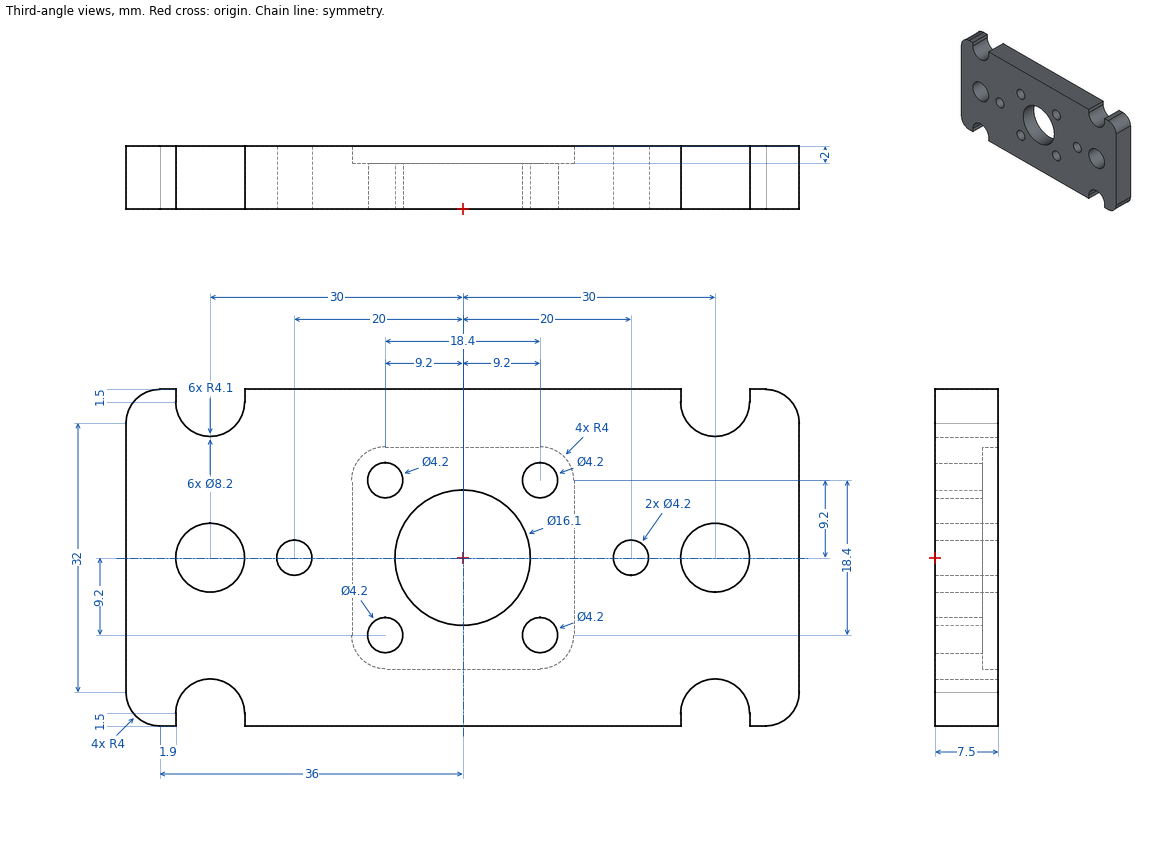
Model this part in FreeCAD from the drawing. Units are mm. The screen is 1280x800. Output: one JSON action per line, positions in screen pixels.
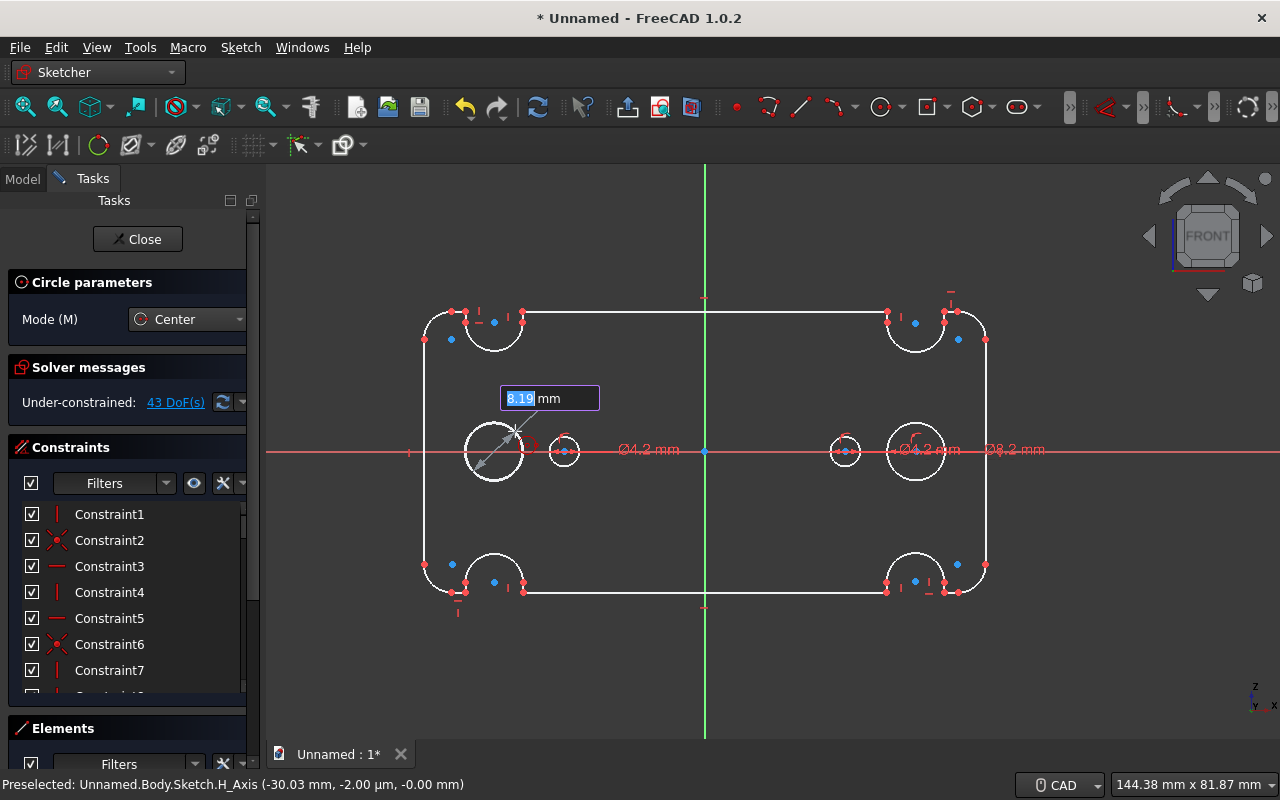
{"action": "type", "text": "8.2"}
{"action": "key", "text": "Return"}
{"action": "key", "text": "Escape"}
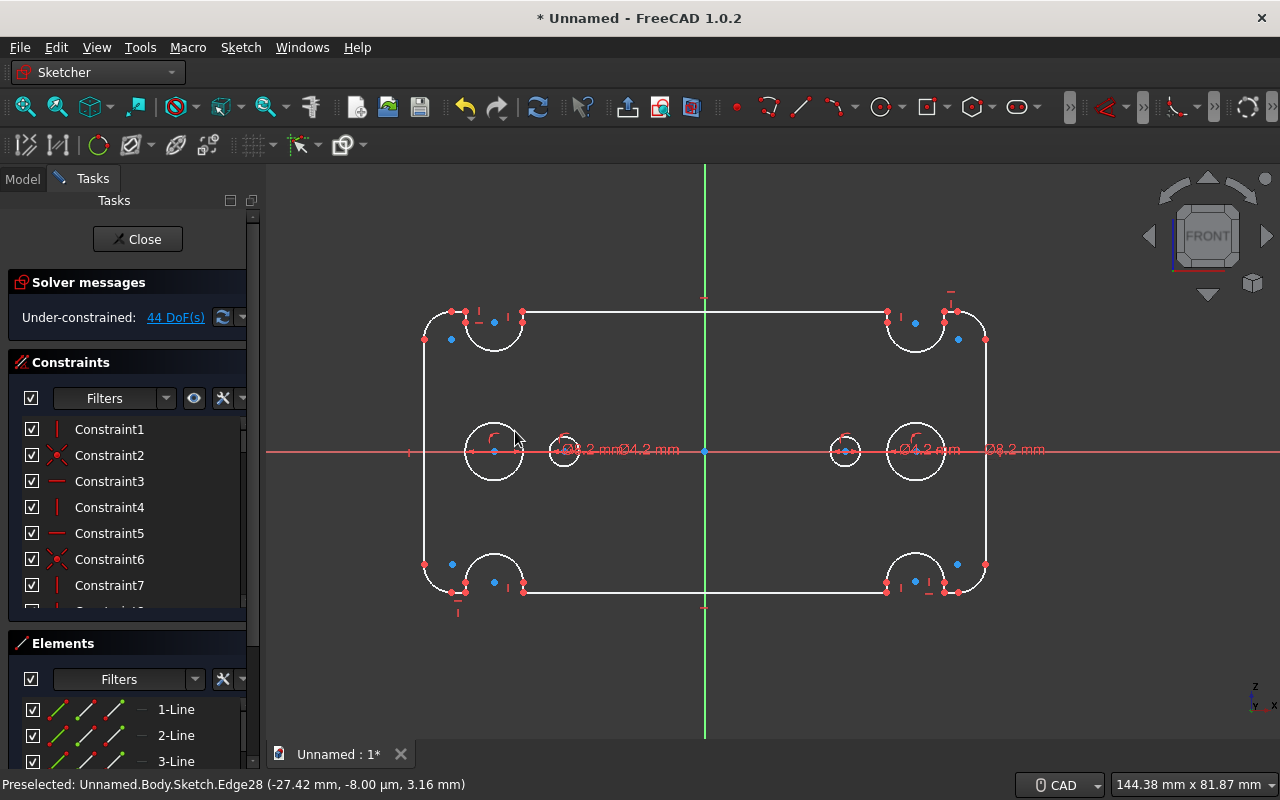
{"action": "scroll", "coordinate": [466, 588], "scroll_direction": "up", "scroll_amount": 6}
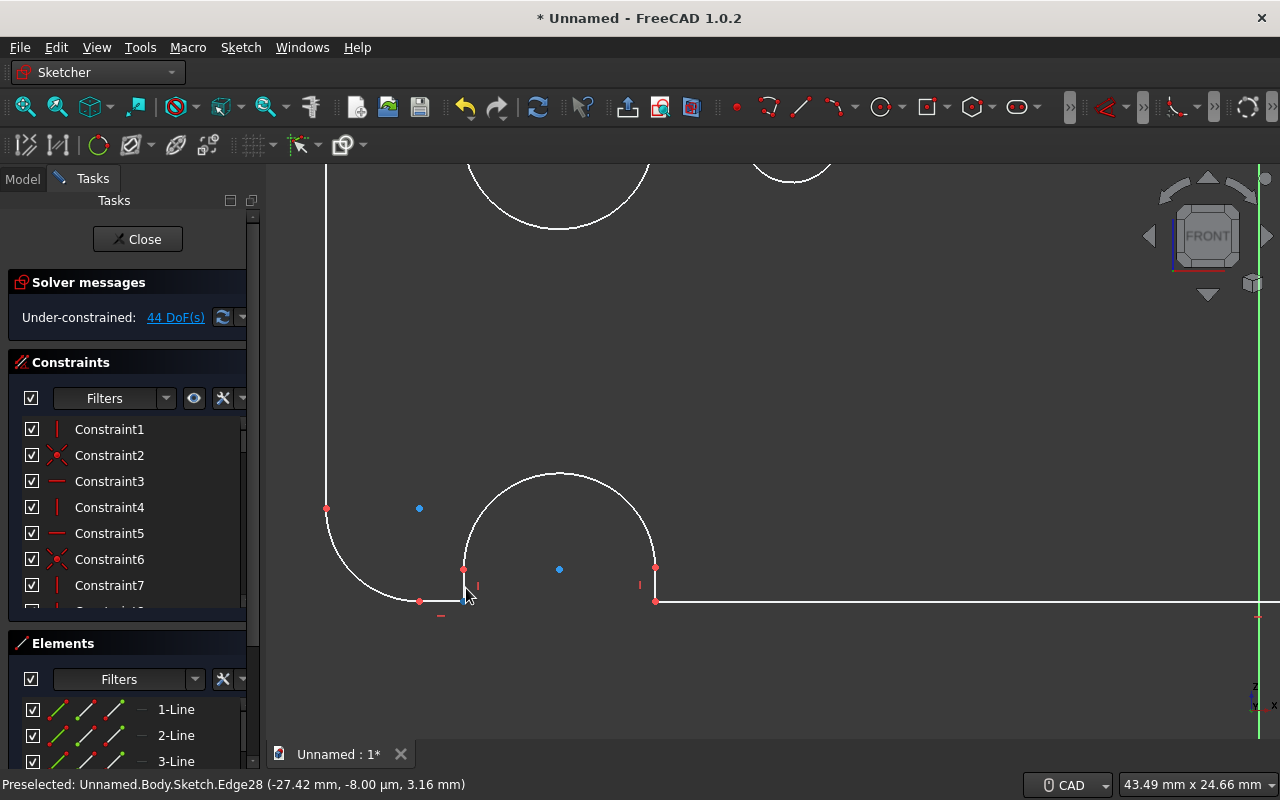
{"action": "left_click", "coordinate": [464, 585]}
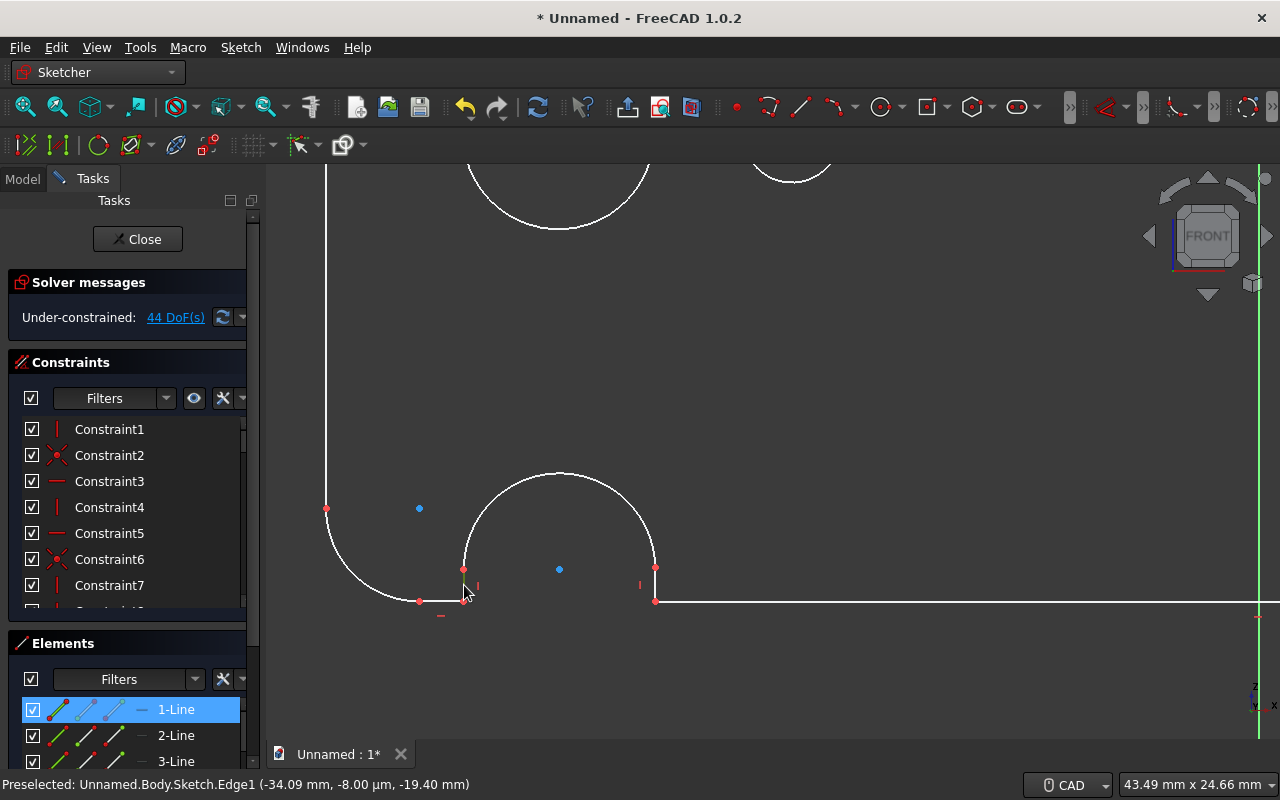
{"action": "scroll", "coordinate": [466, 589], "scroll_direction": "down", "scroll_amount": 6}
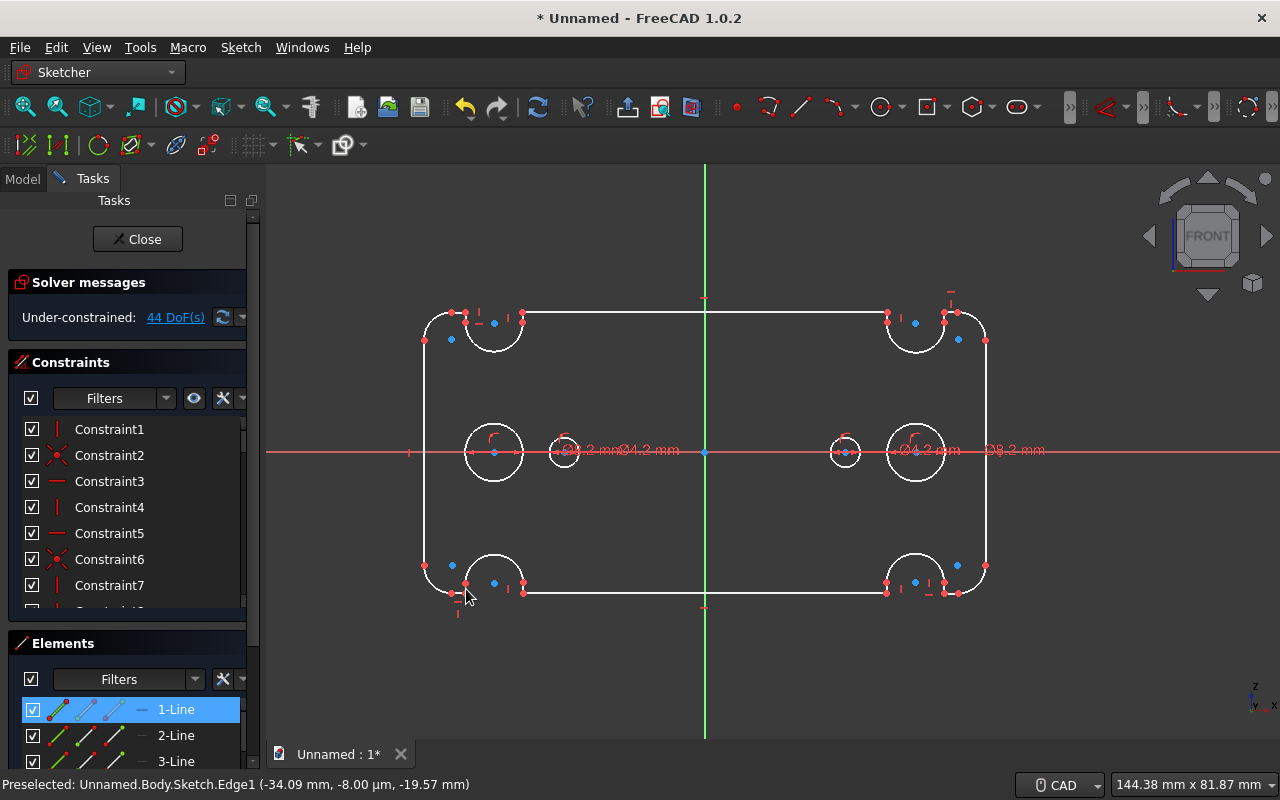
{"action": "left_click", "coordinate": [511, 560]}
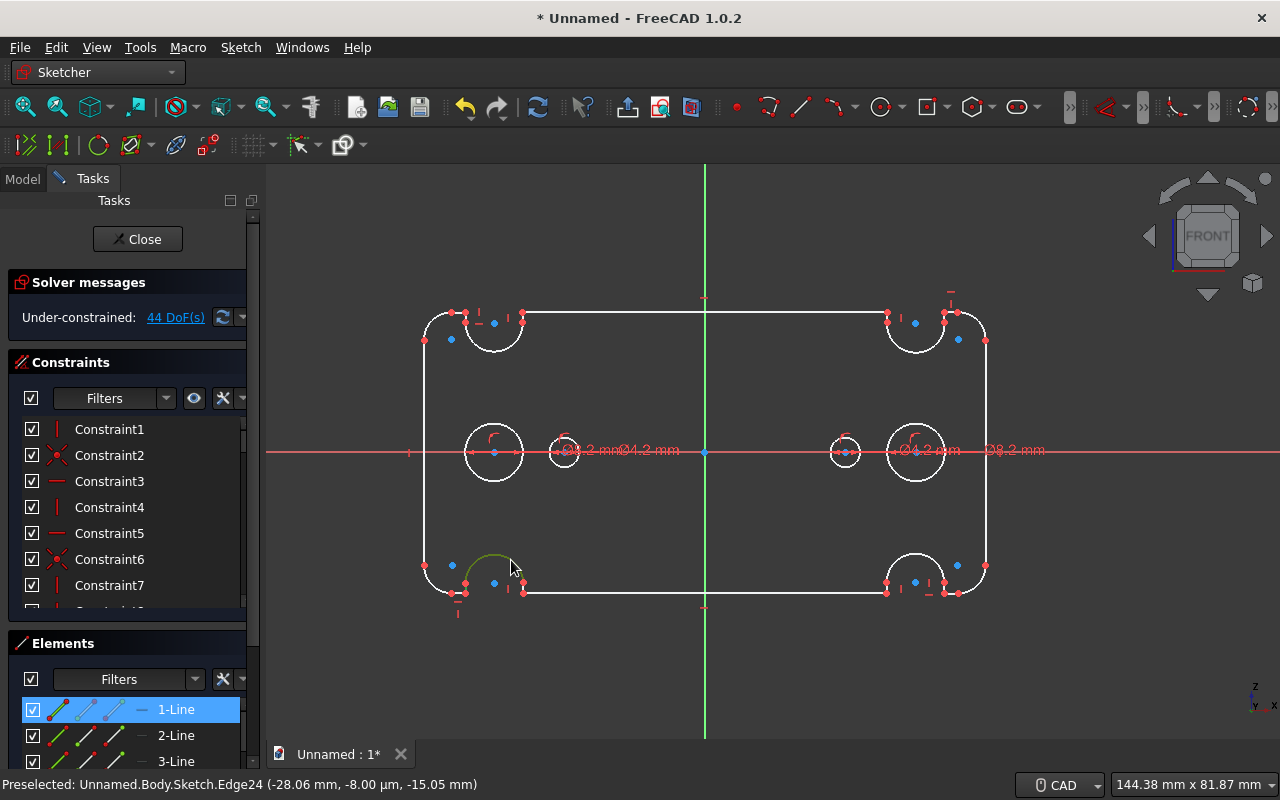
{"action": "key", "text": "t"}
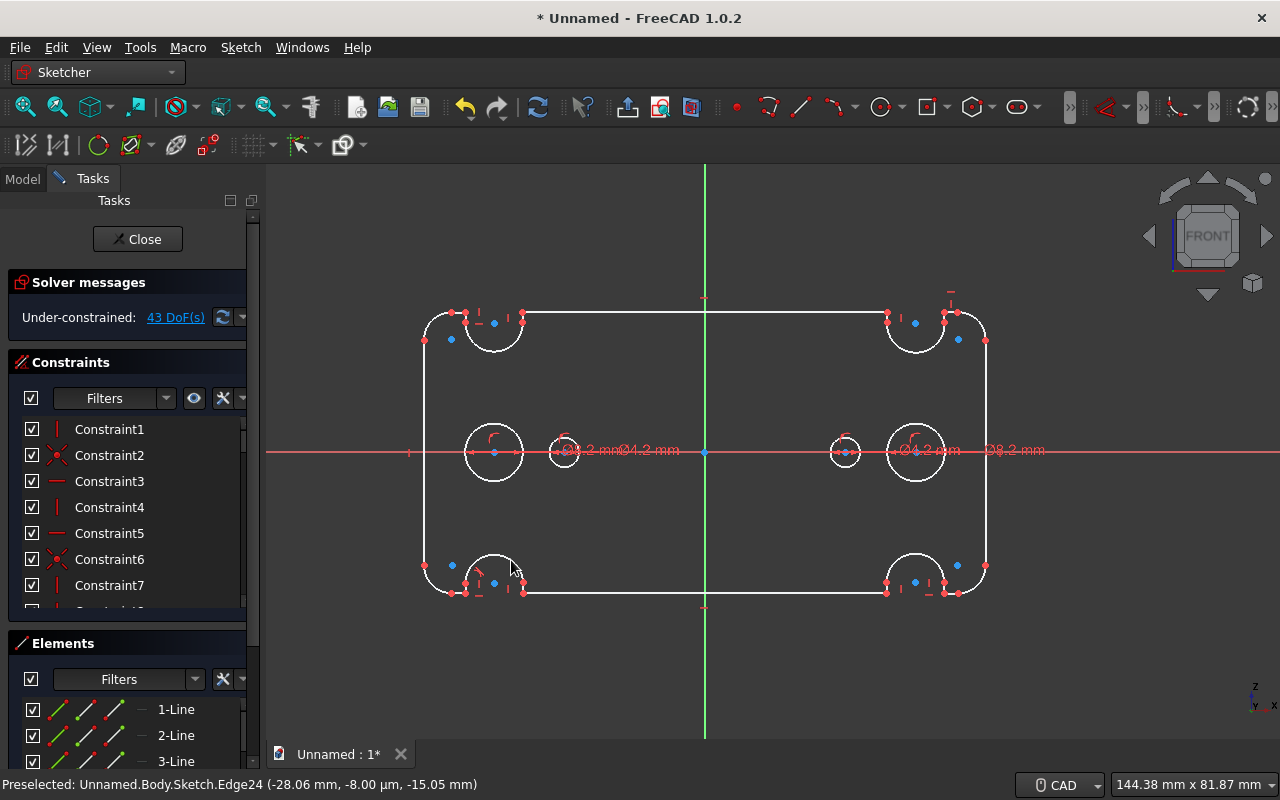
{"action": "scroll", "coordinate": [459, 593], "scroll_direction": "up", "scroll_amount": 4}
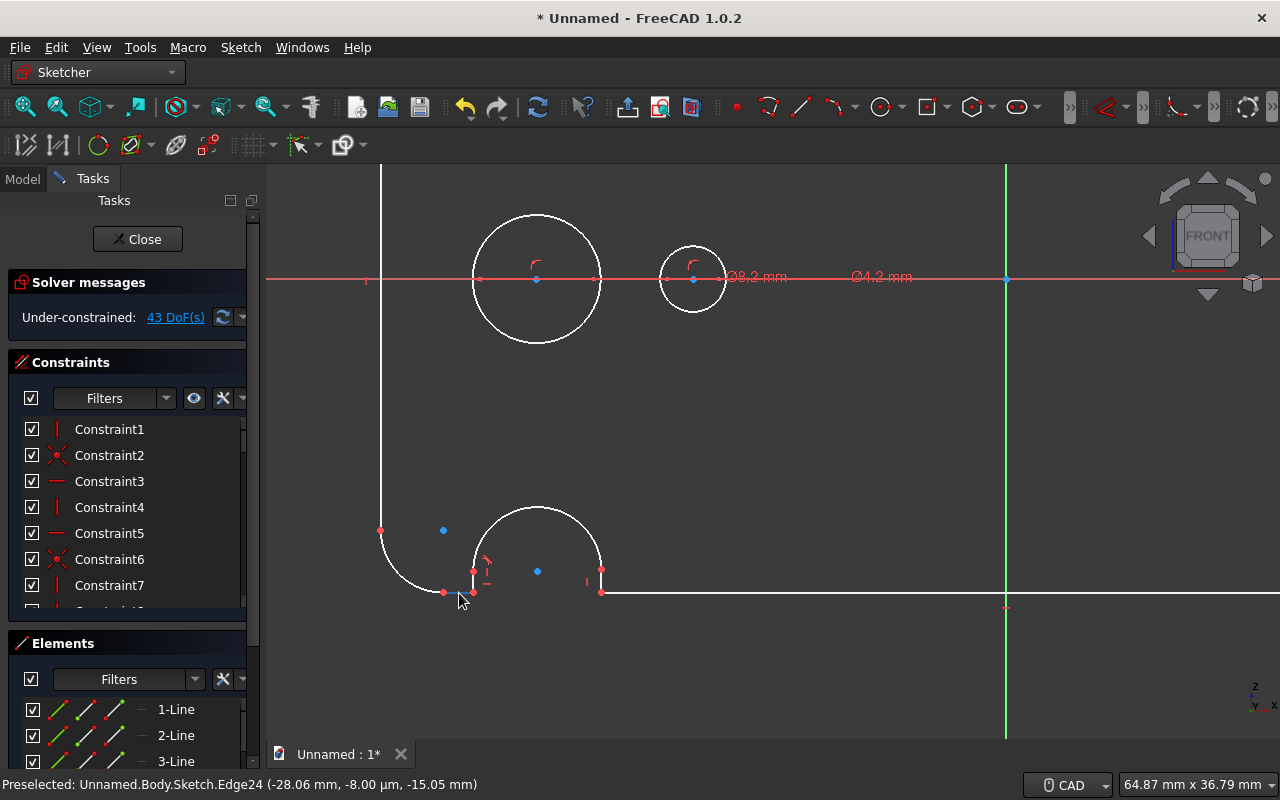
{"action": "left_click", "coordinate": [458, 593]}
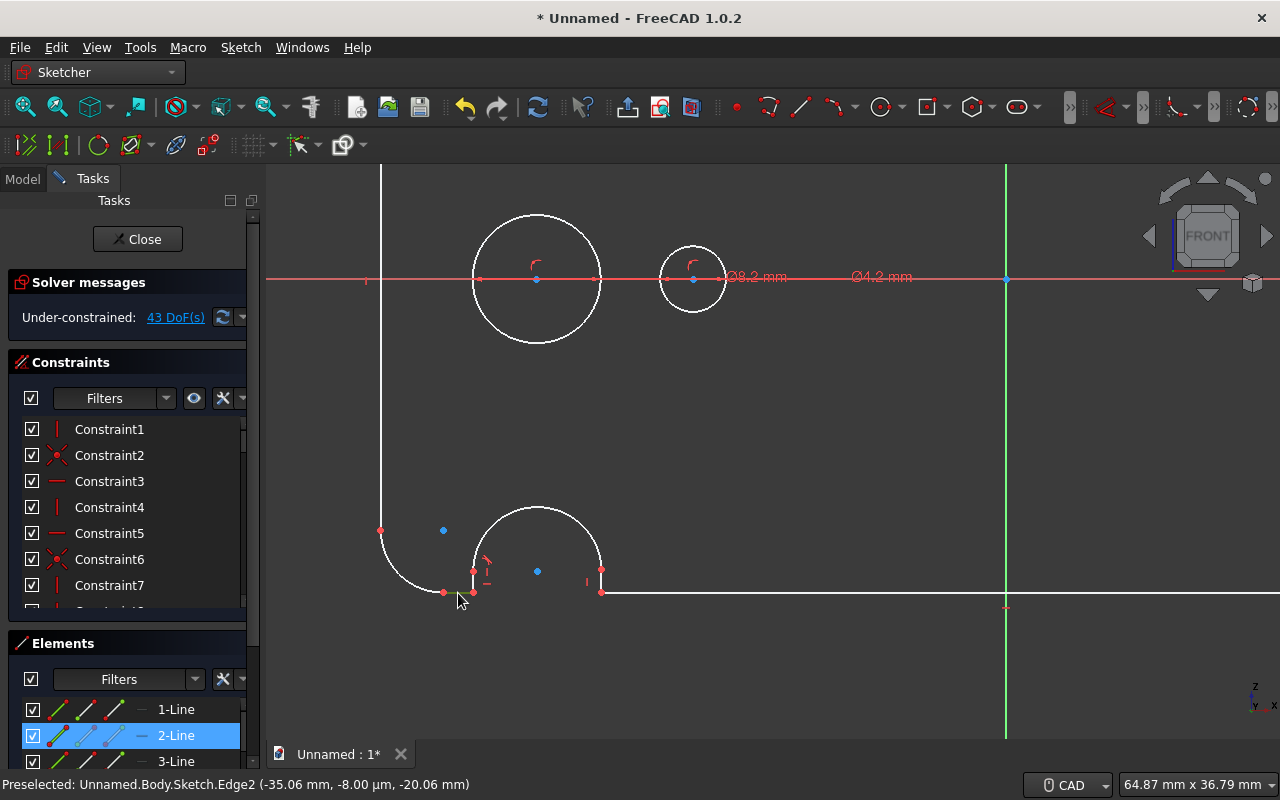
{"action": "left_click", "coordinate": [388, 559]}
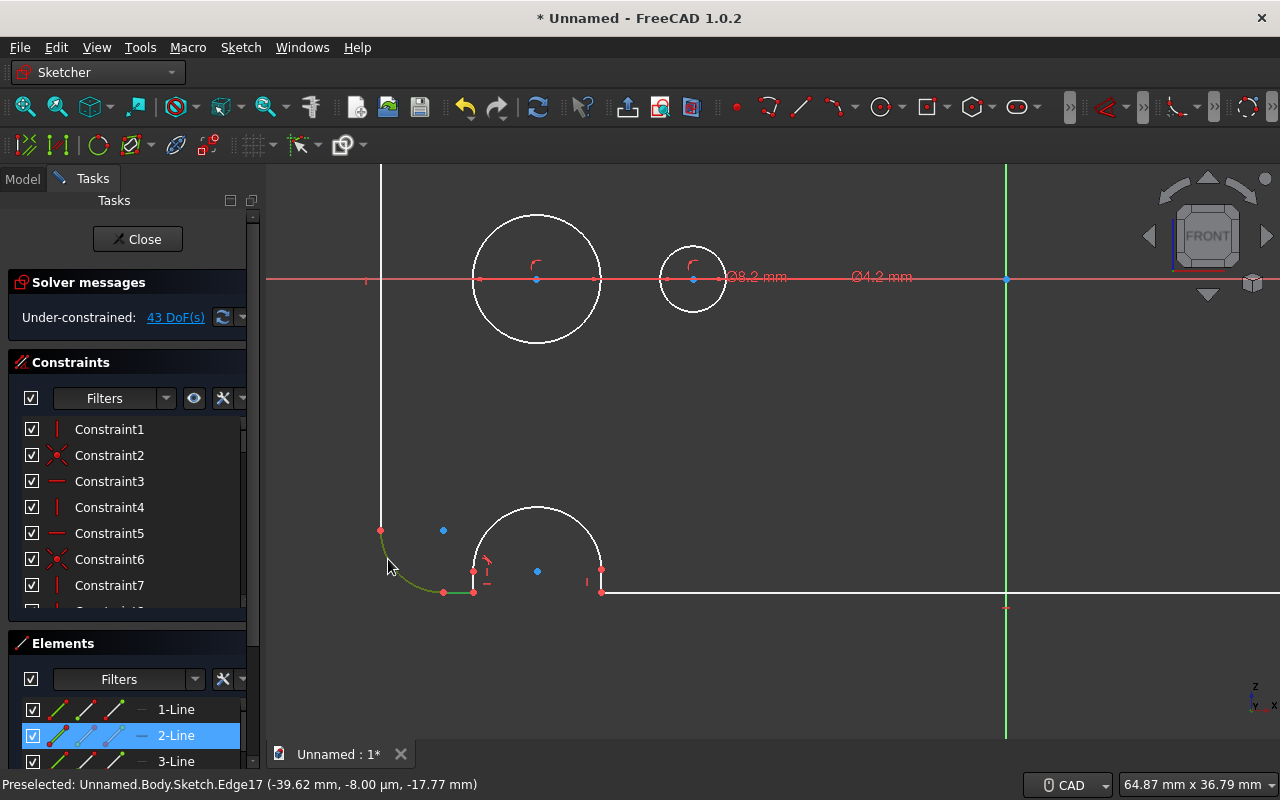
{"action": "key", "text": "t"}